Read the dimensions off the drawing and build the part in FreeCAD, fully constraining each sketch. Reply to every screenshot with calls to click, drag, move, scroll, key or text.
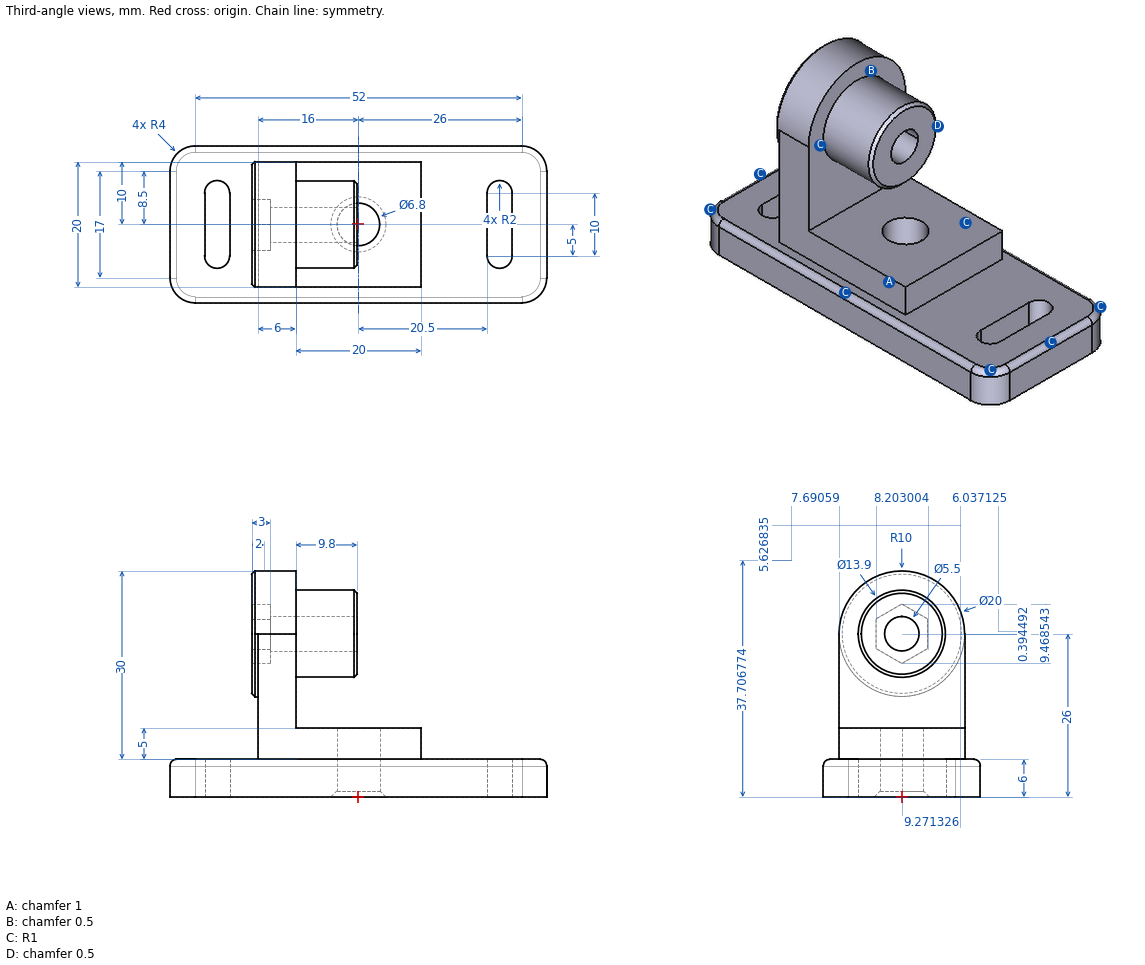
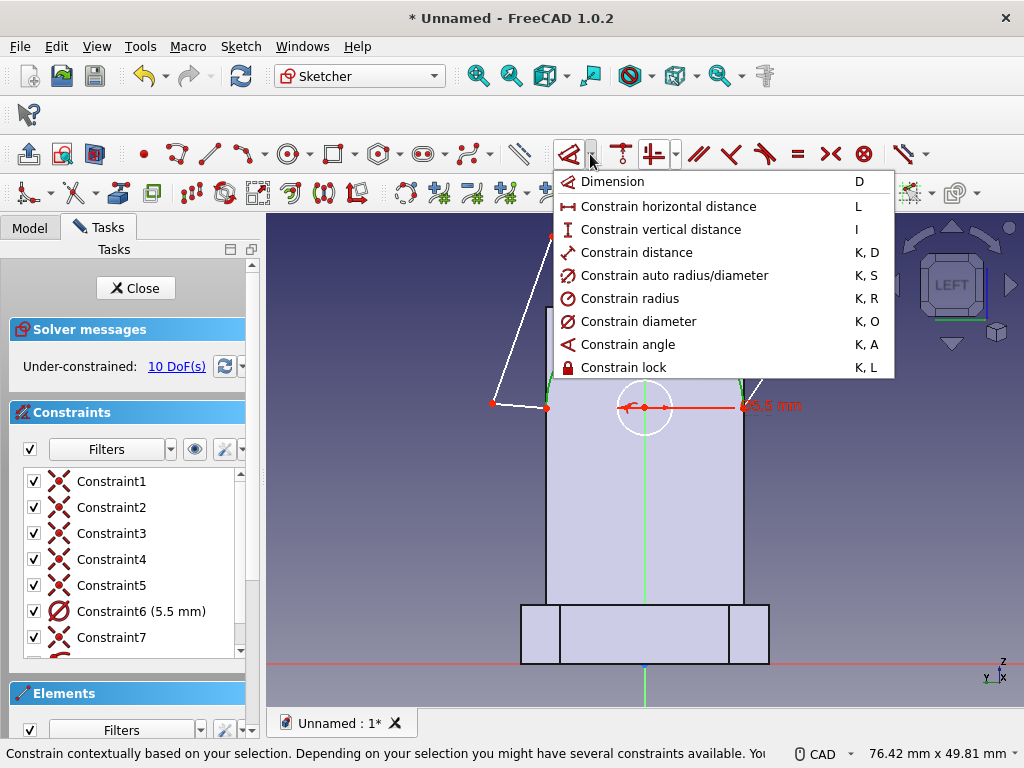
click(724, 298)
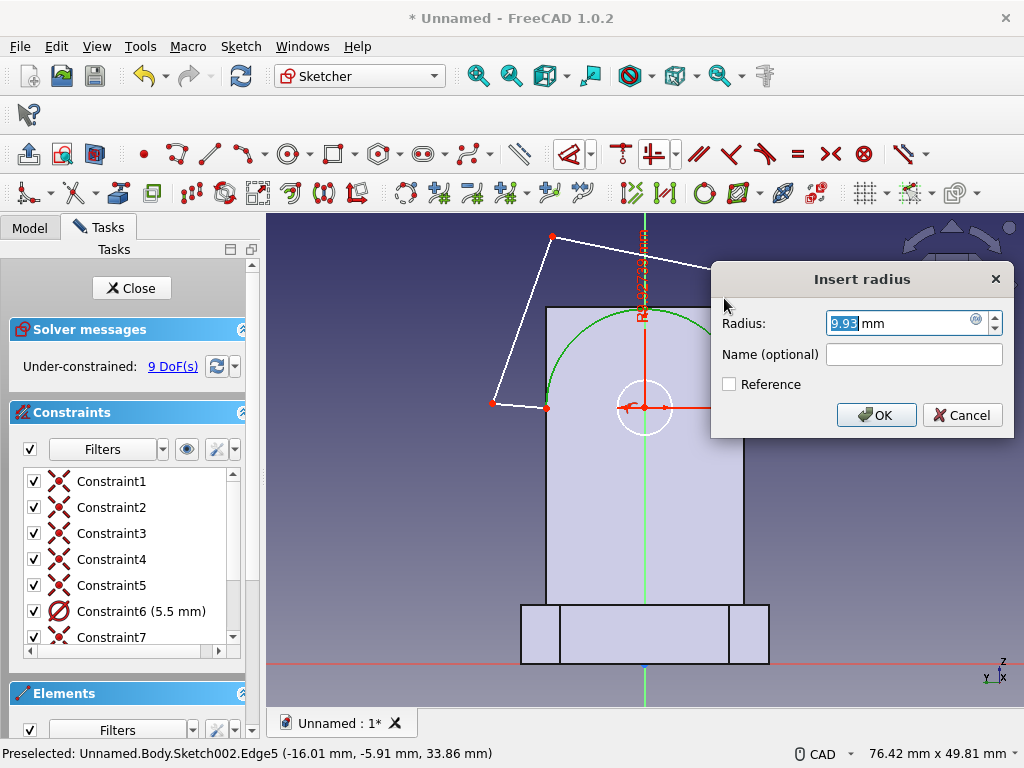
text(10)
key(Return)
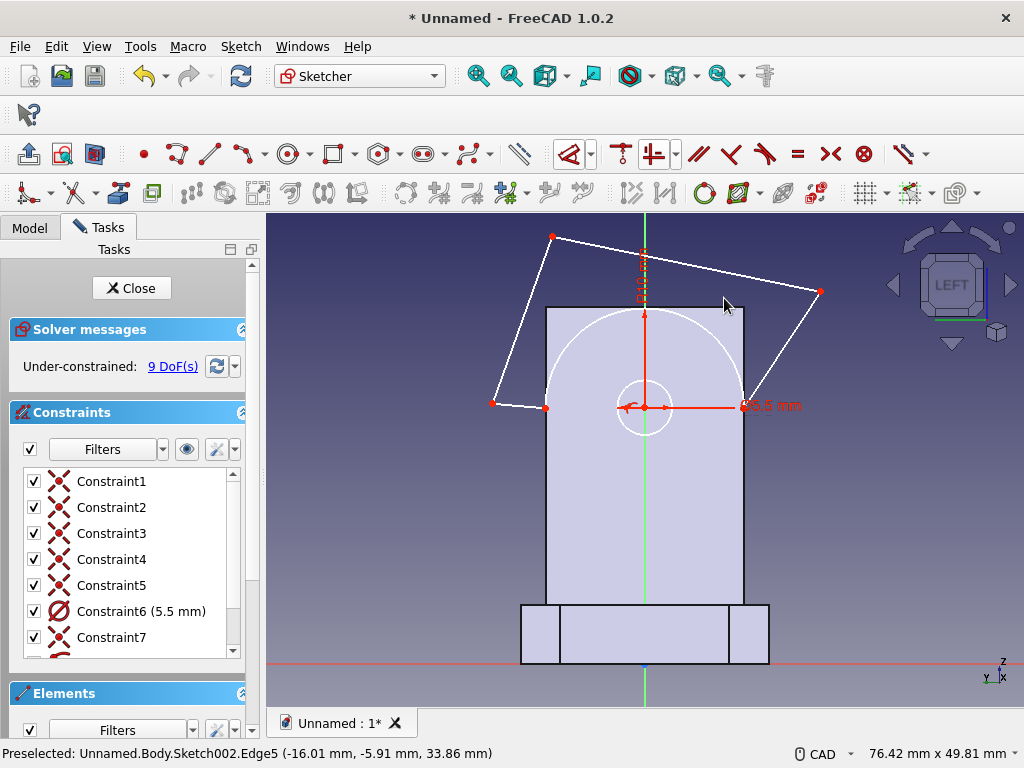
click(645, 408)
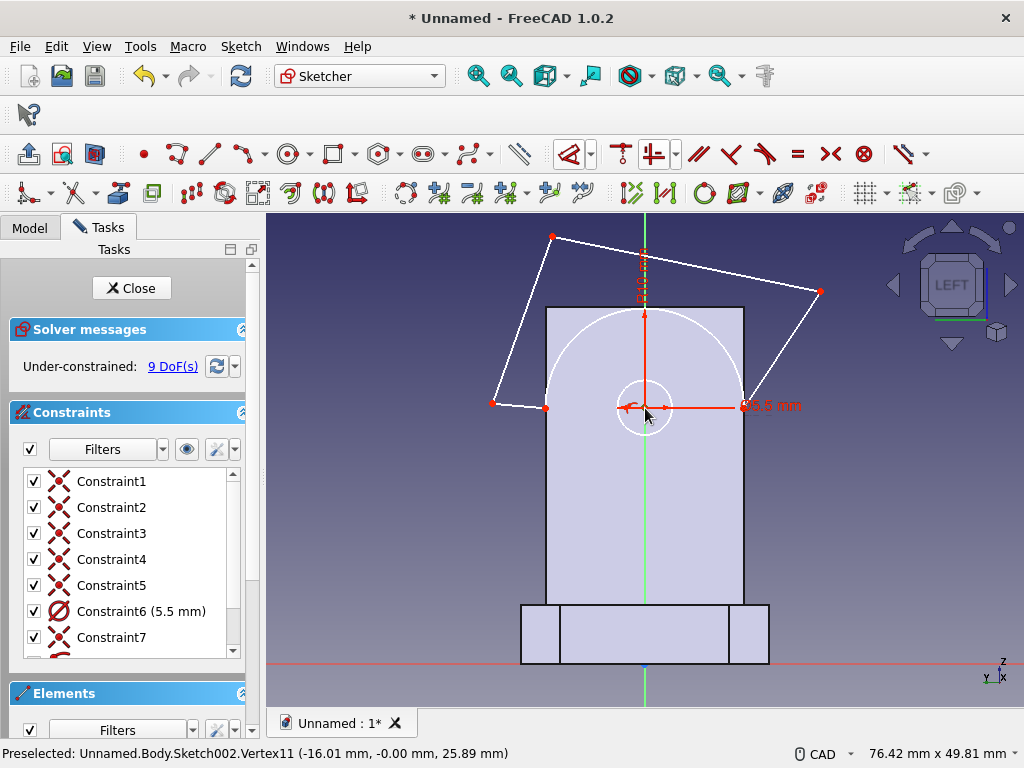
key(i)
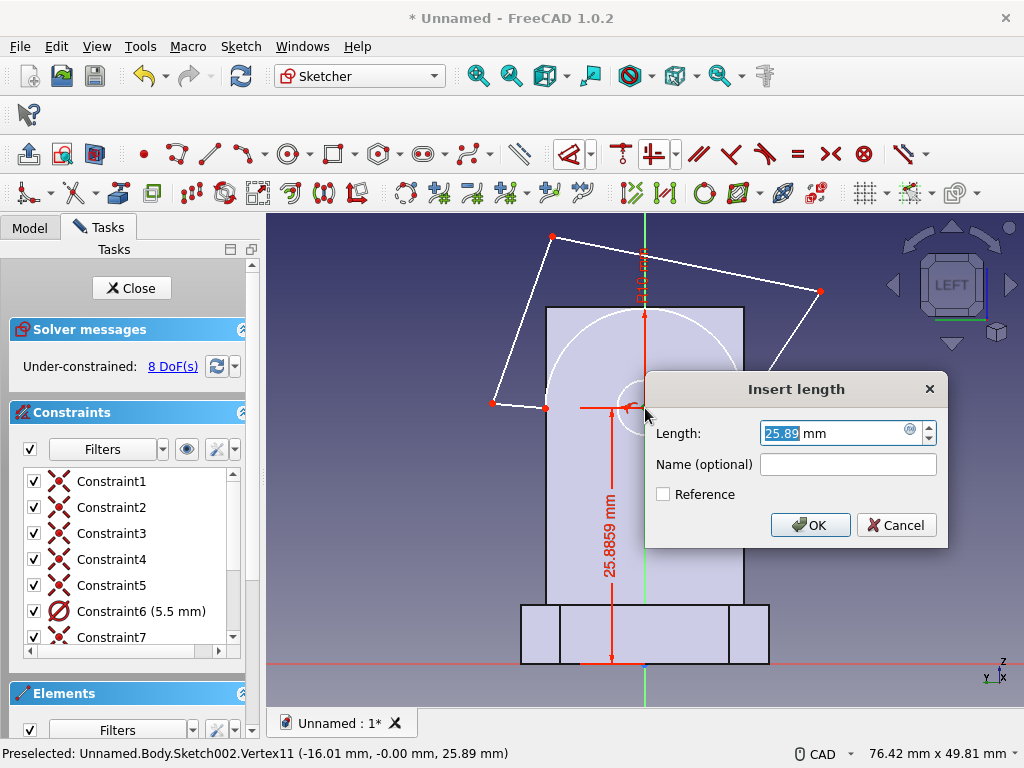
text(26)
key(Return)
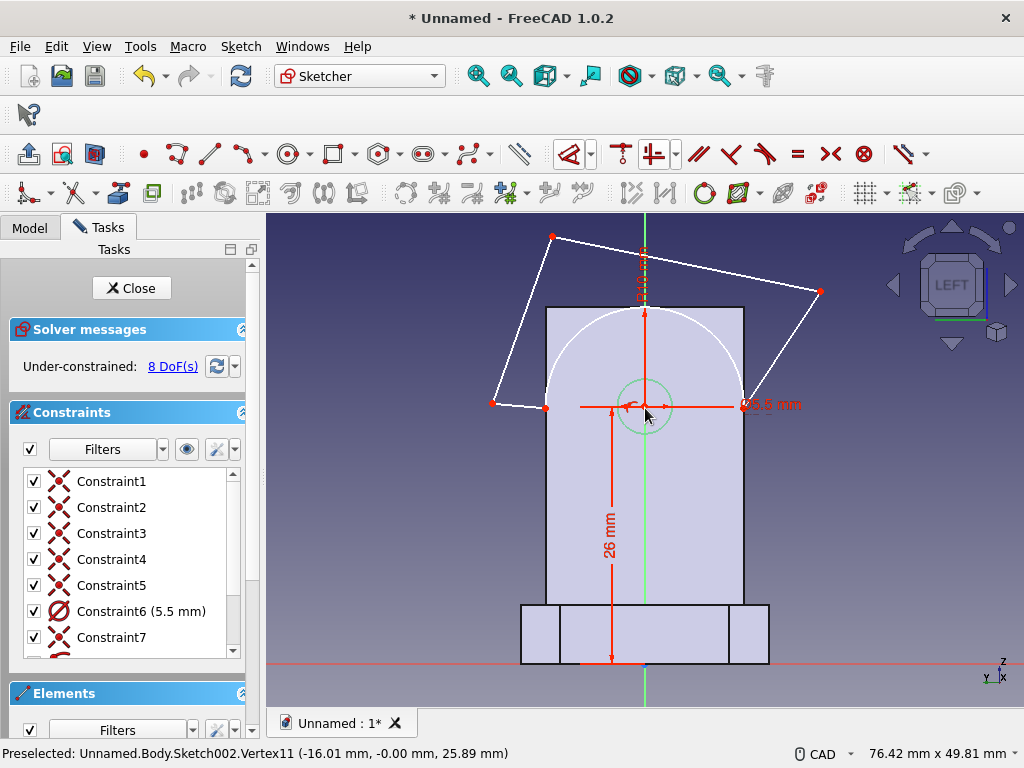
click(744, 408)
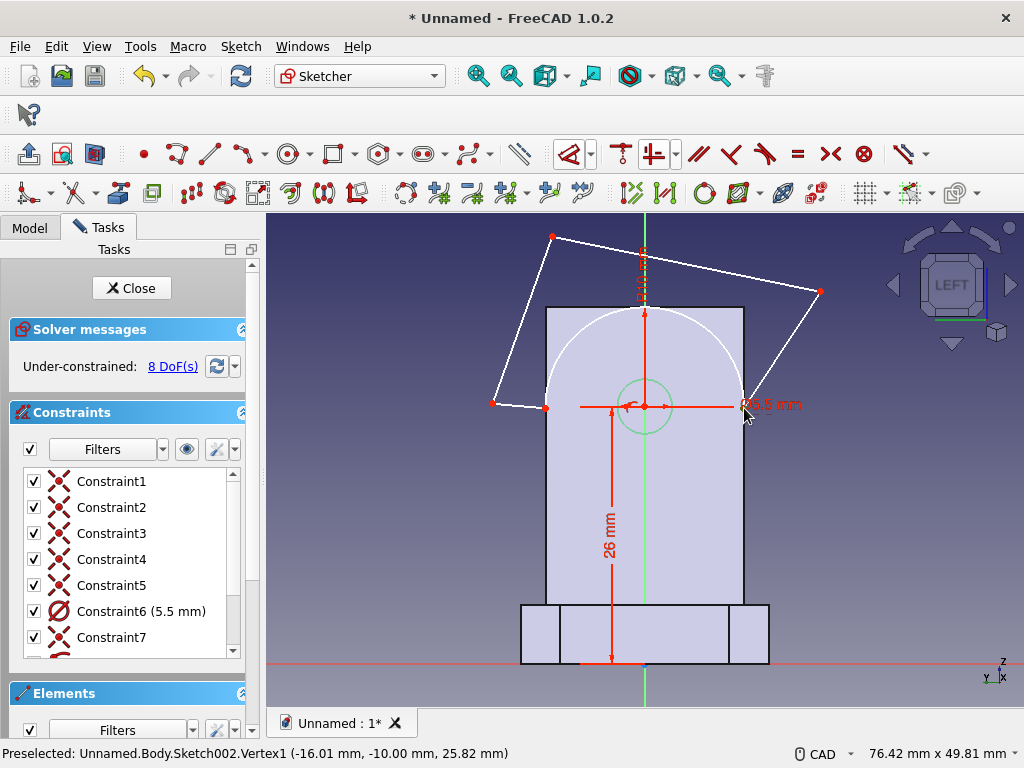
click(590, 154)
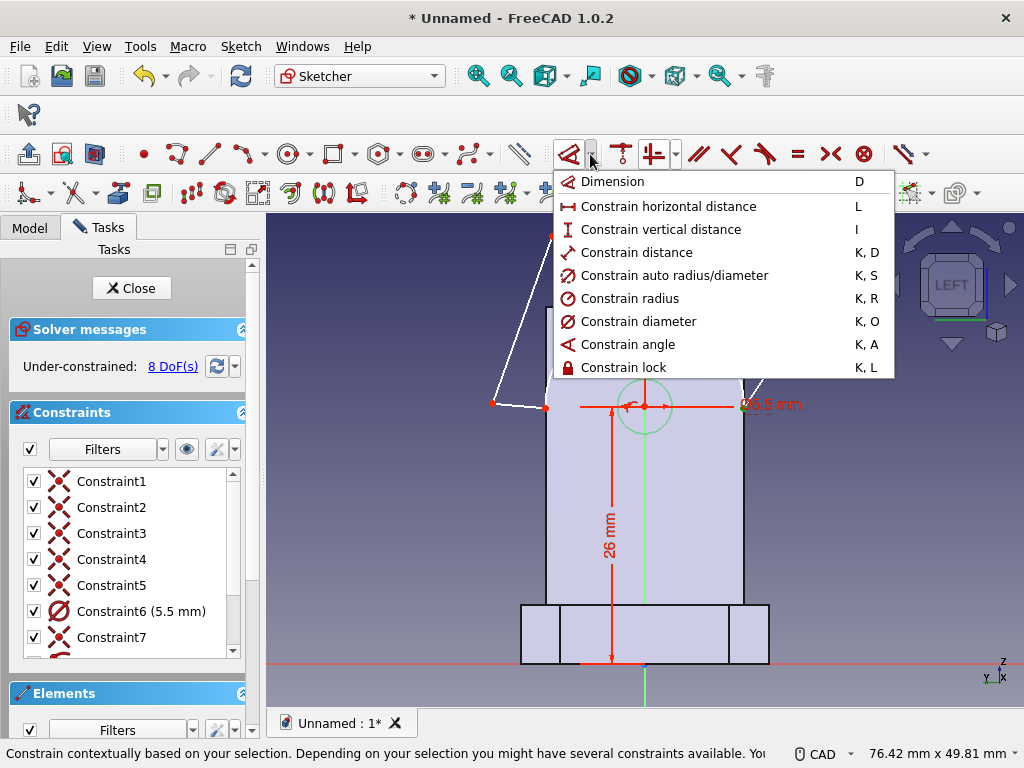
click(724, 230)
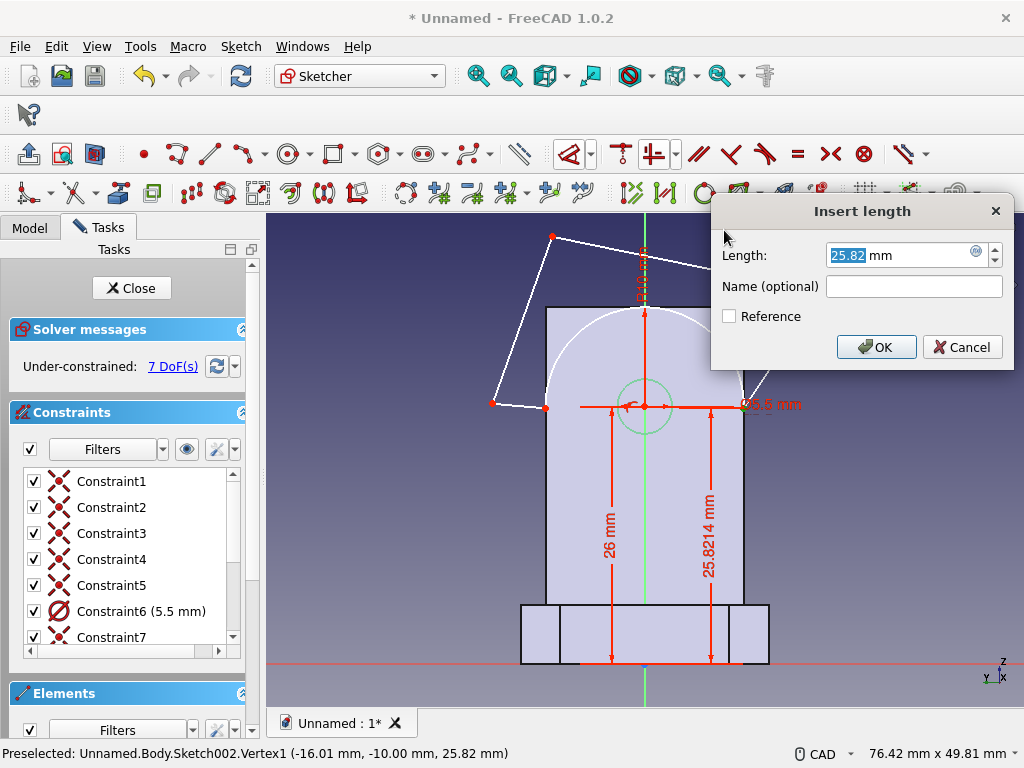
text(26)
key(Return)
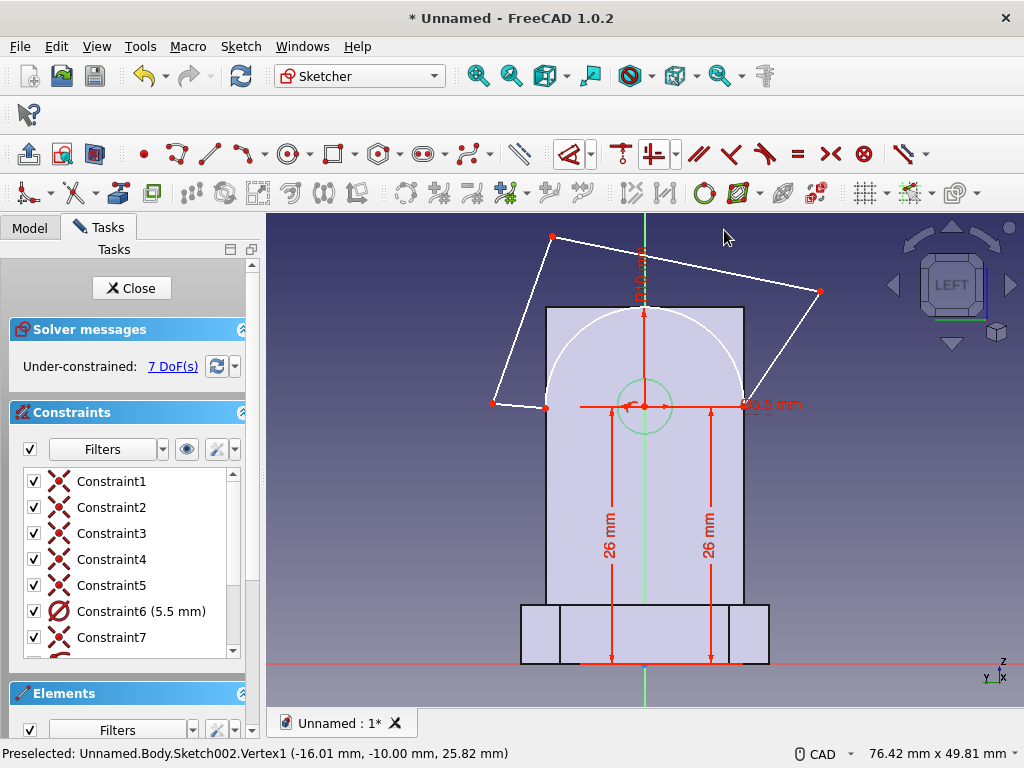
click(546, 408)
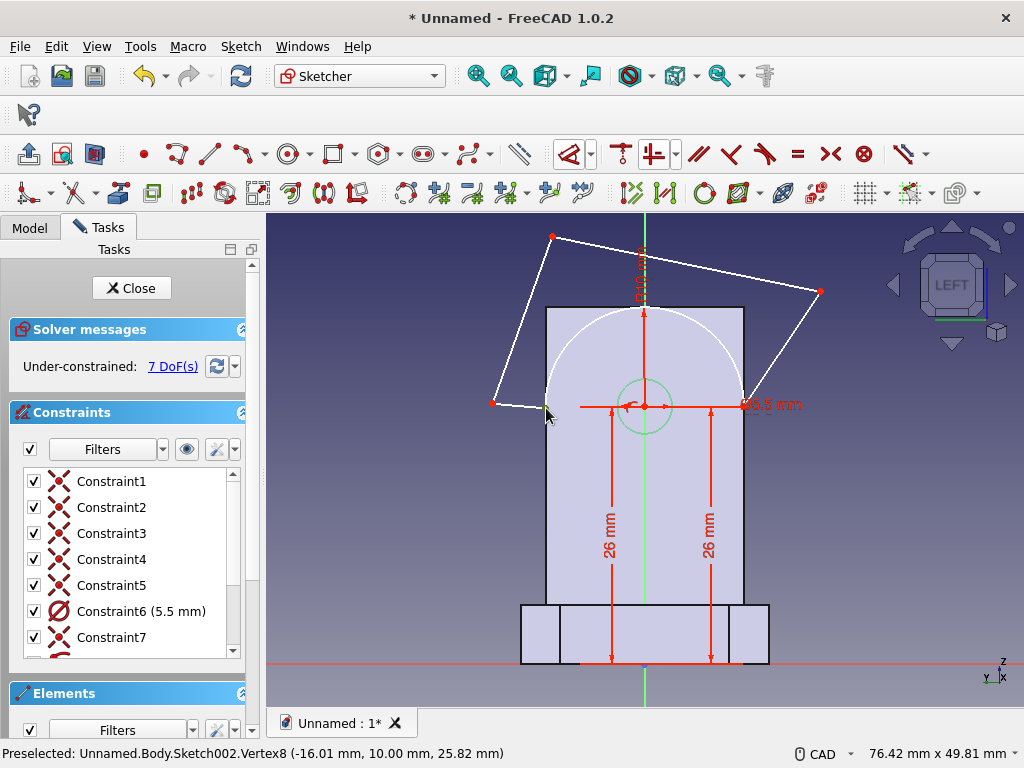
key(i)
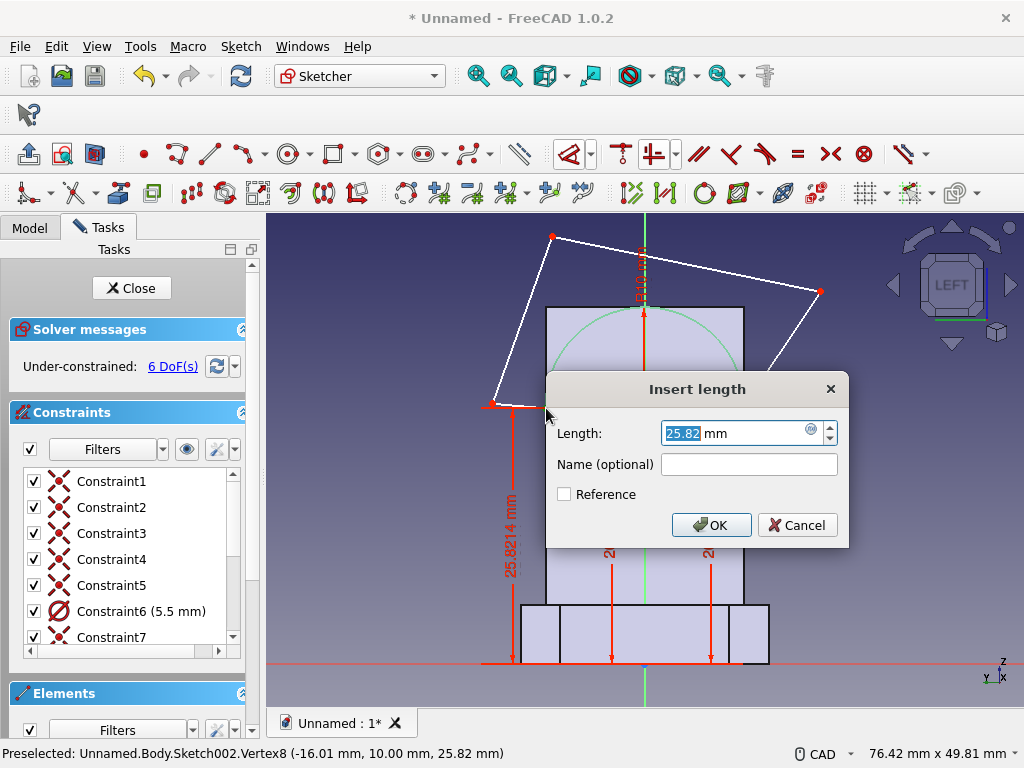
text(26)
key(Return)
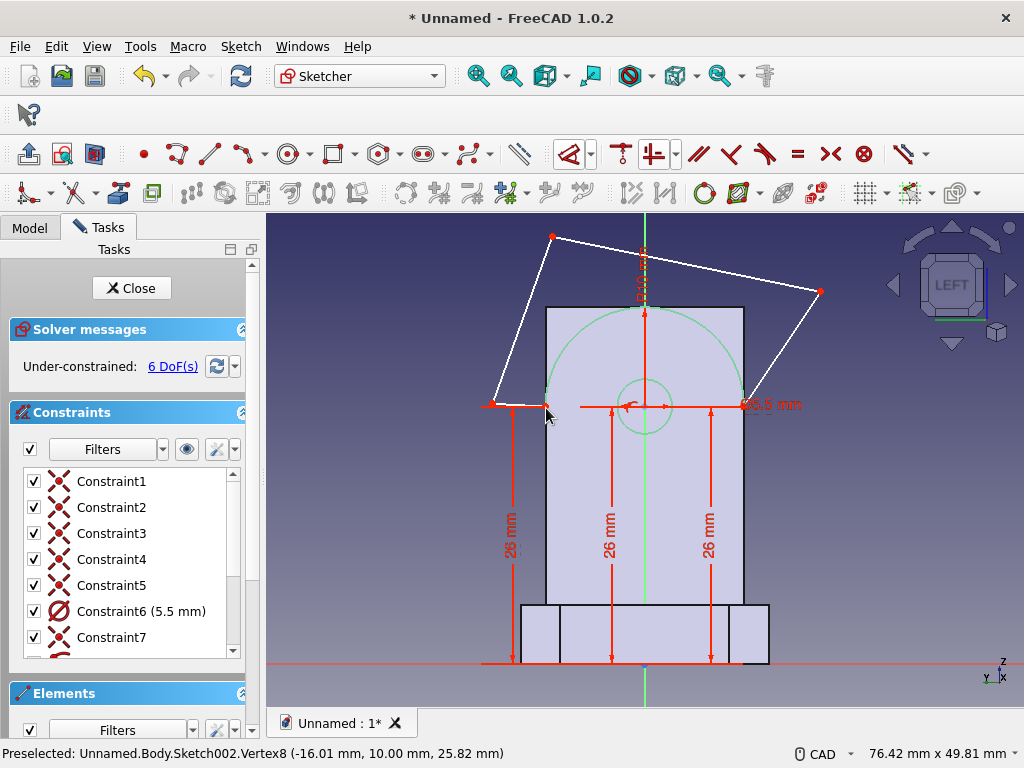
click(767, 372)